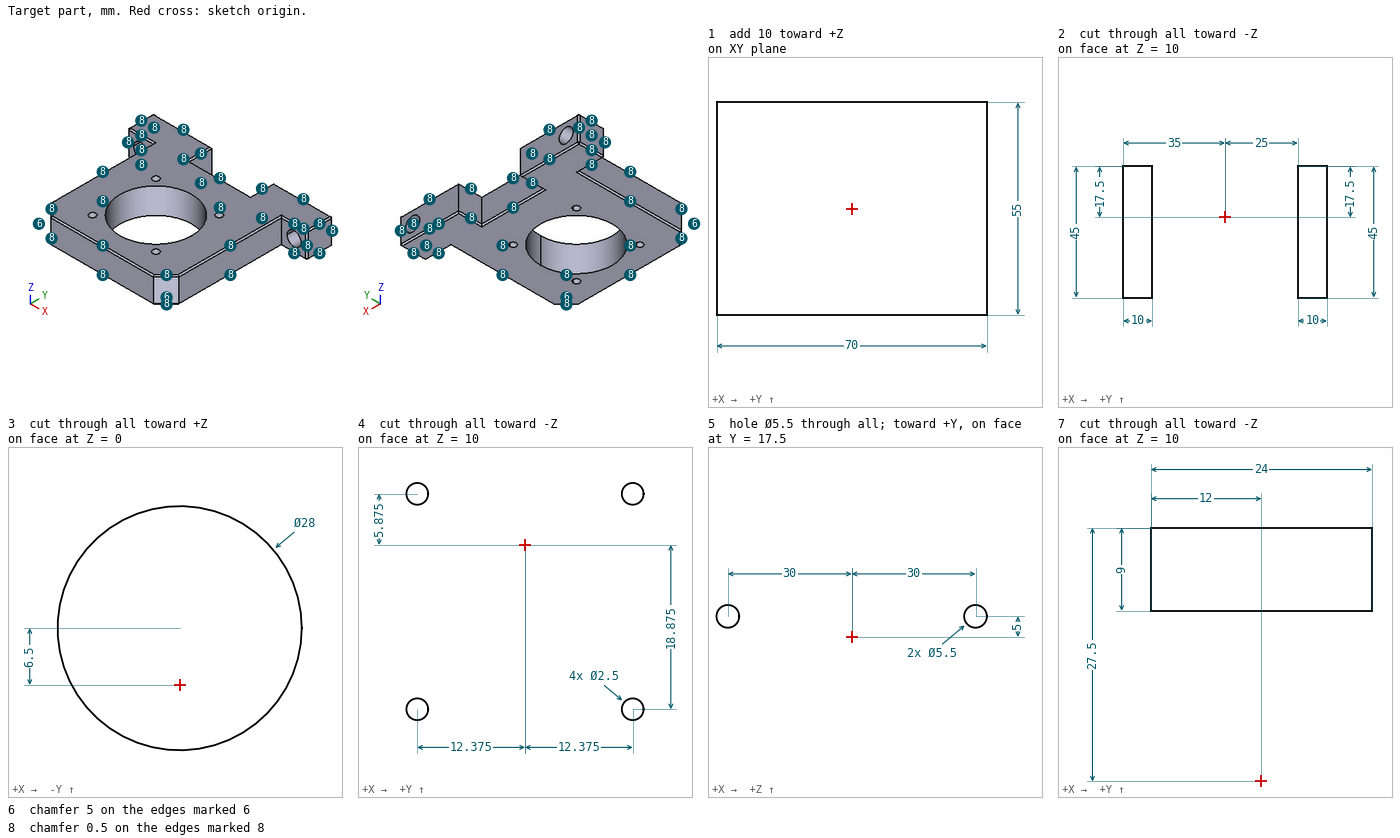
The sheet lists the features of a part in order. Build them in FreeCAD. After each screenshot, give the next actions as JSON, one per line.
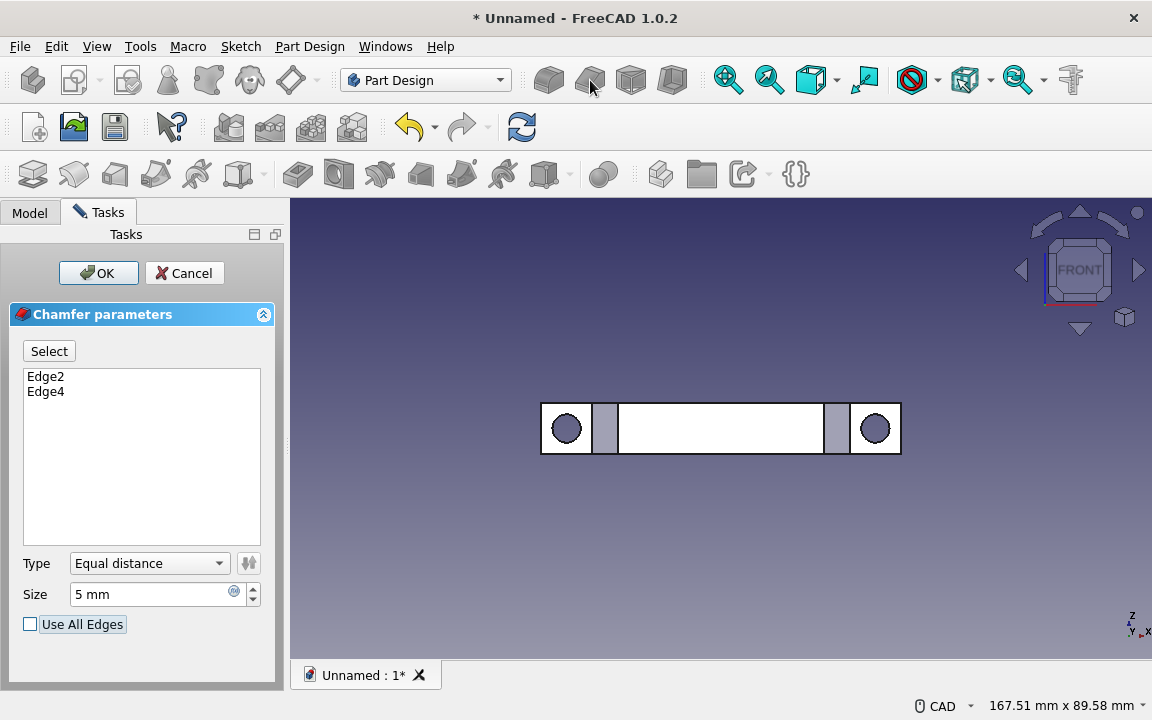
{"action": "left_click", "coordinate": [99, 273]}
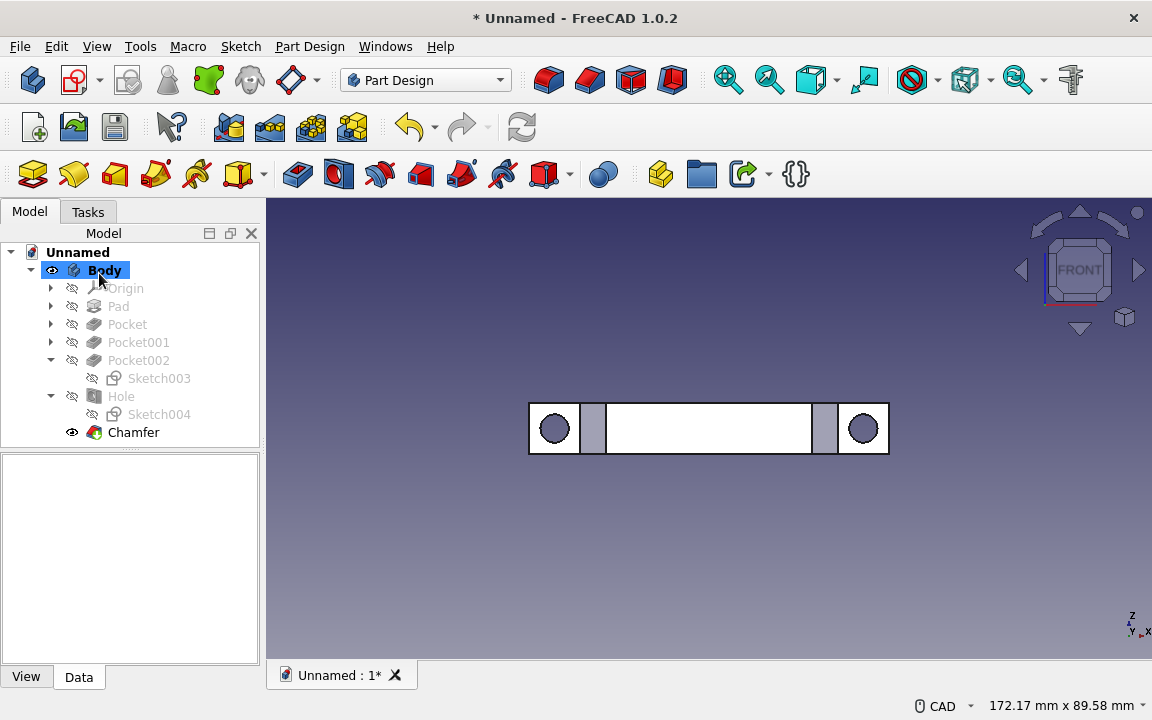
{"action": "key", "text": "v f"}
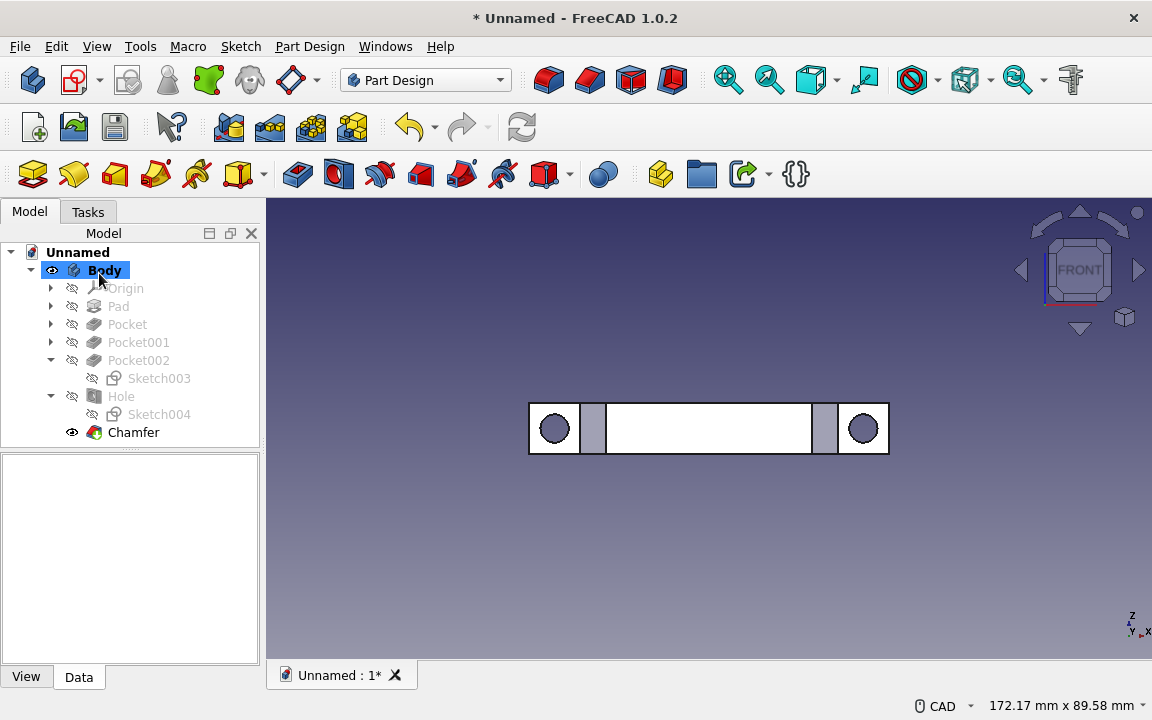
{"action": "key", "text": "0"}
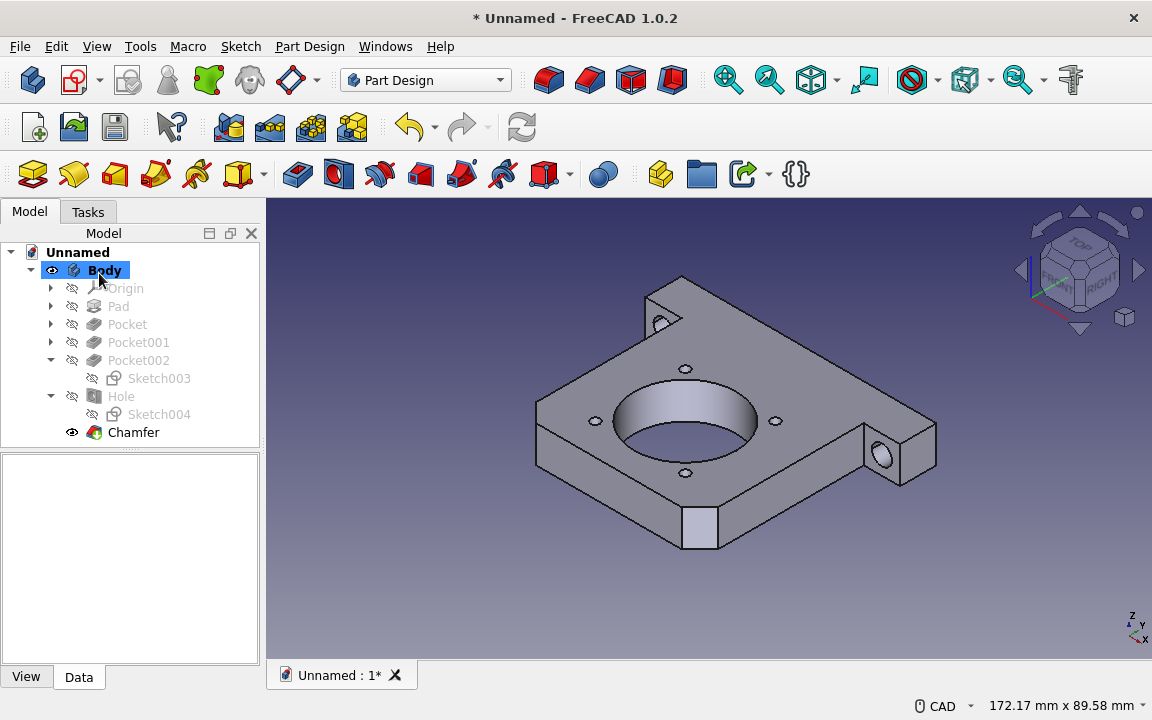
{"action": "left_click", "coordinate": [803, 394]}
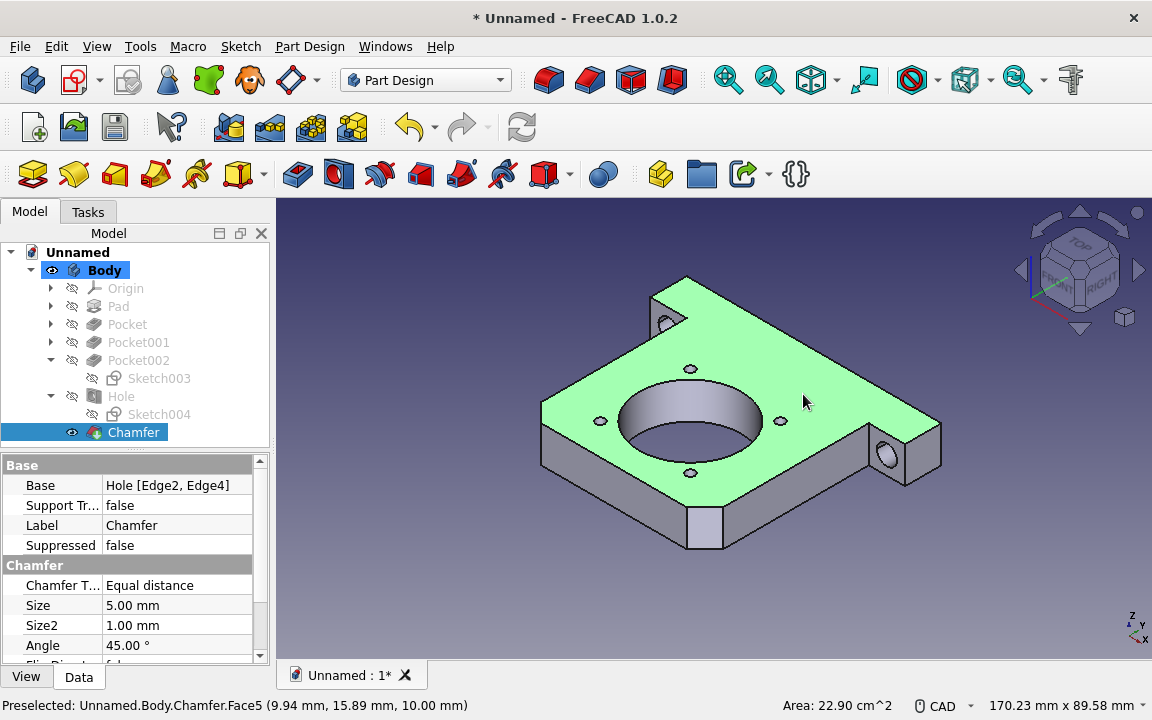
{"action": "left_click", "coordinate": [74, 80]}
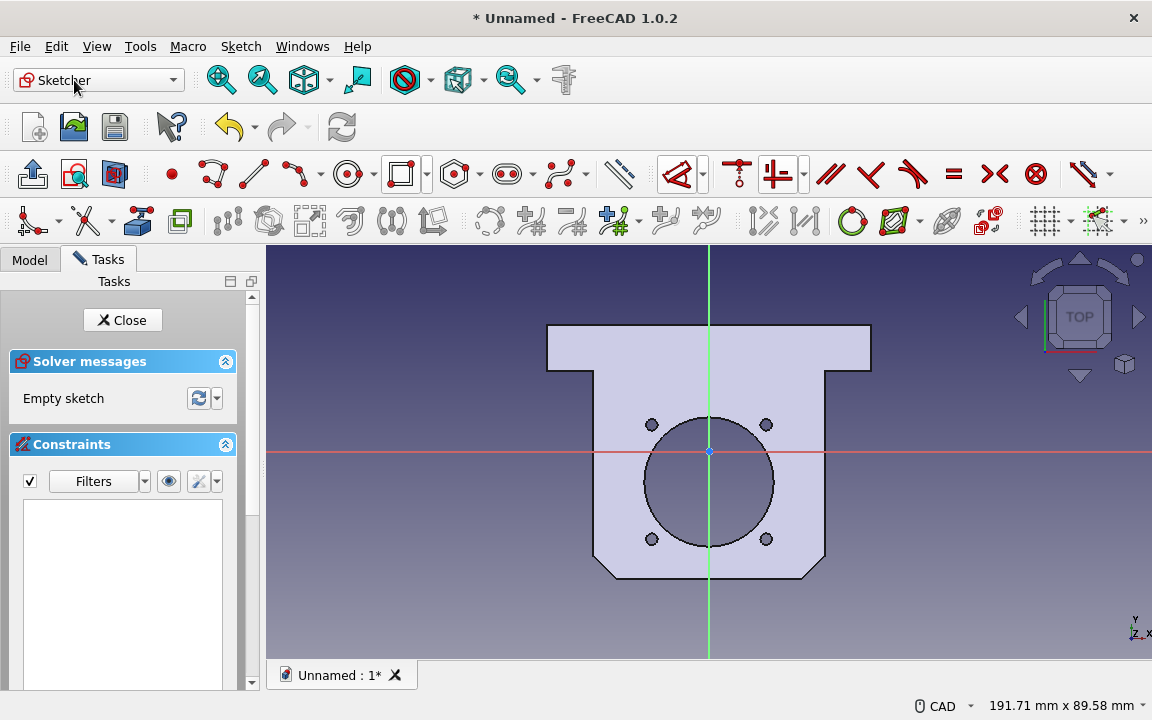
{"action": "scroll", "coordinate": [792, 311], "scroll_direction": "up", "scroll_amount": 3}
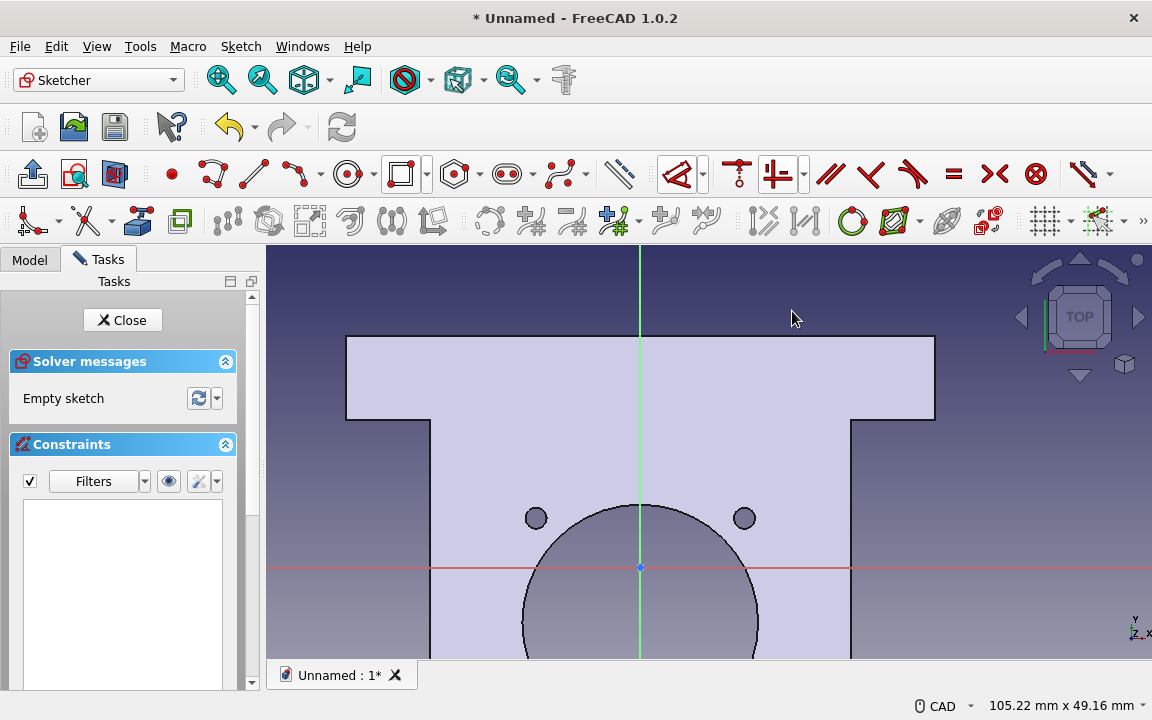
{"action": "left_click", "coordinate": [400, 174]}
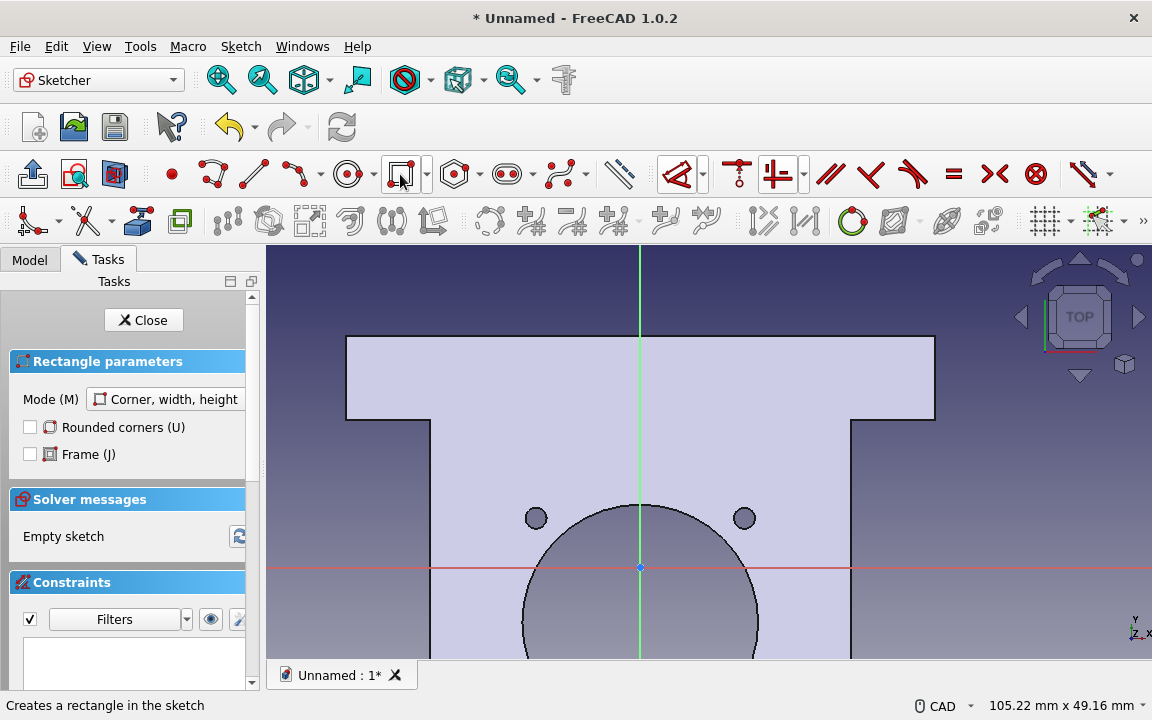
{"action": "left_click", "coordinate": [539, 336]}
{"action": "left_click", "coordinate": [741, 412]}
{"action": "key", "text": "Escape"}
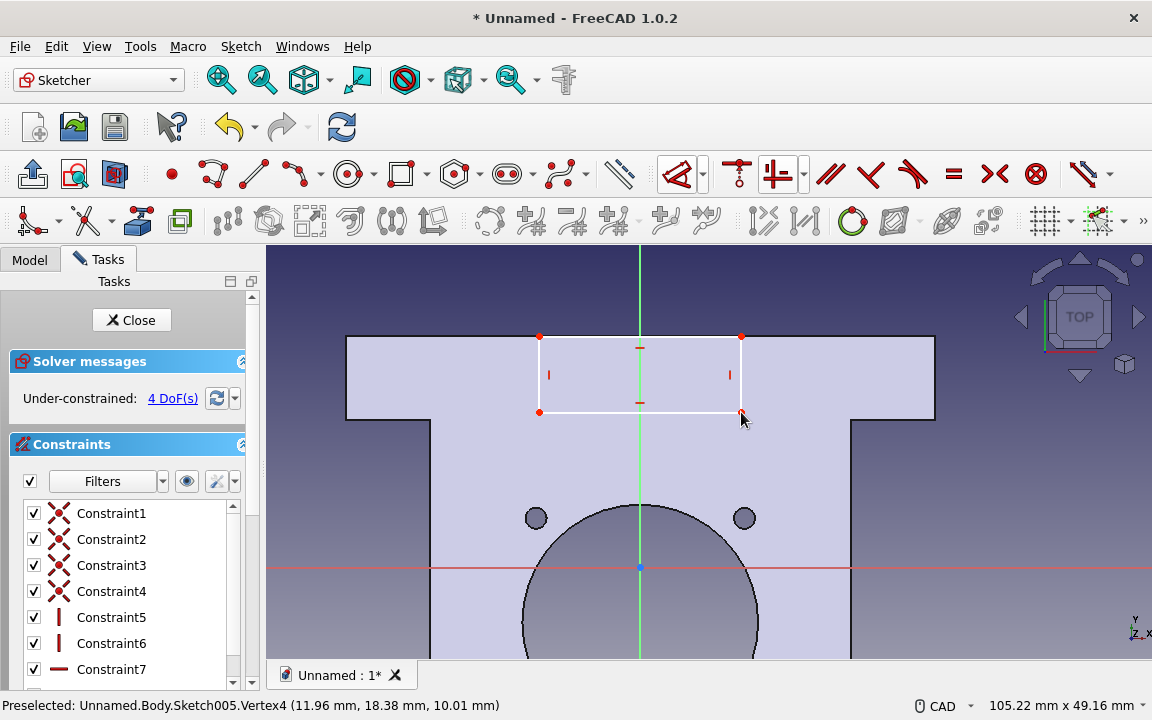
{"action": "left_click", "coordinate": [539, 360]}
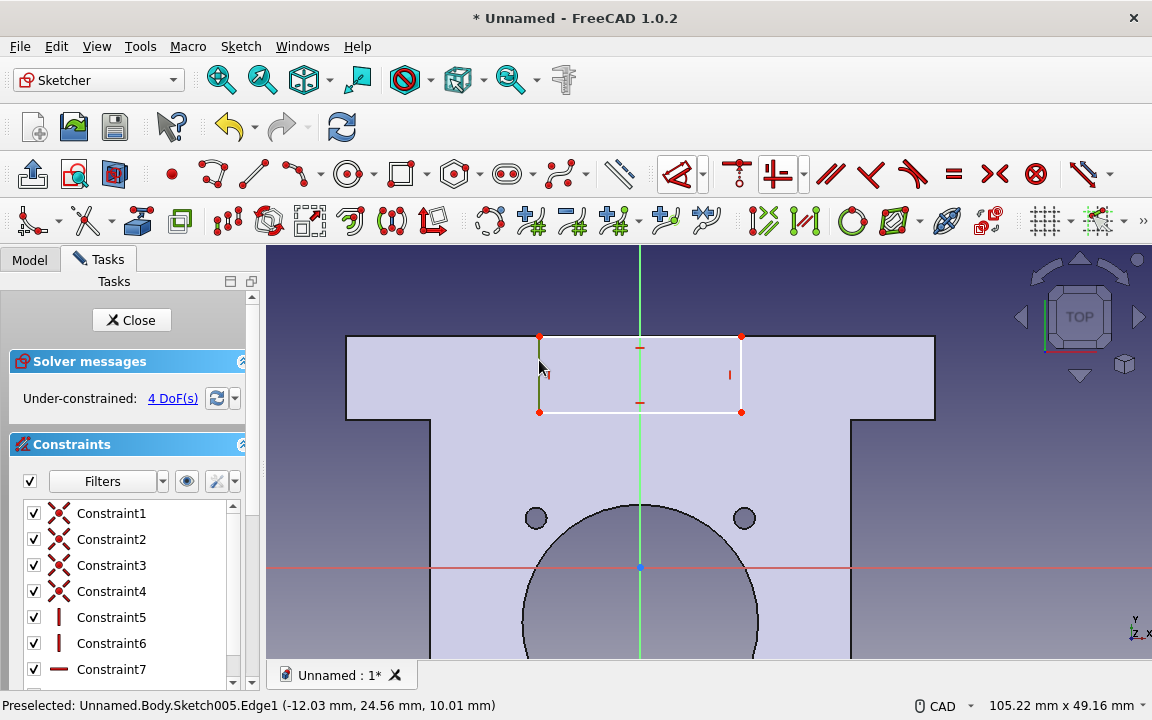
{"action": "key", "text": "i"}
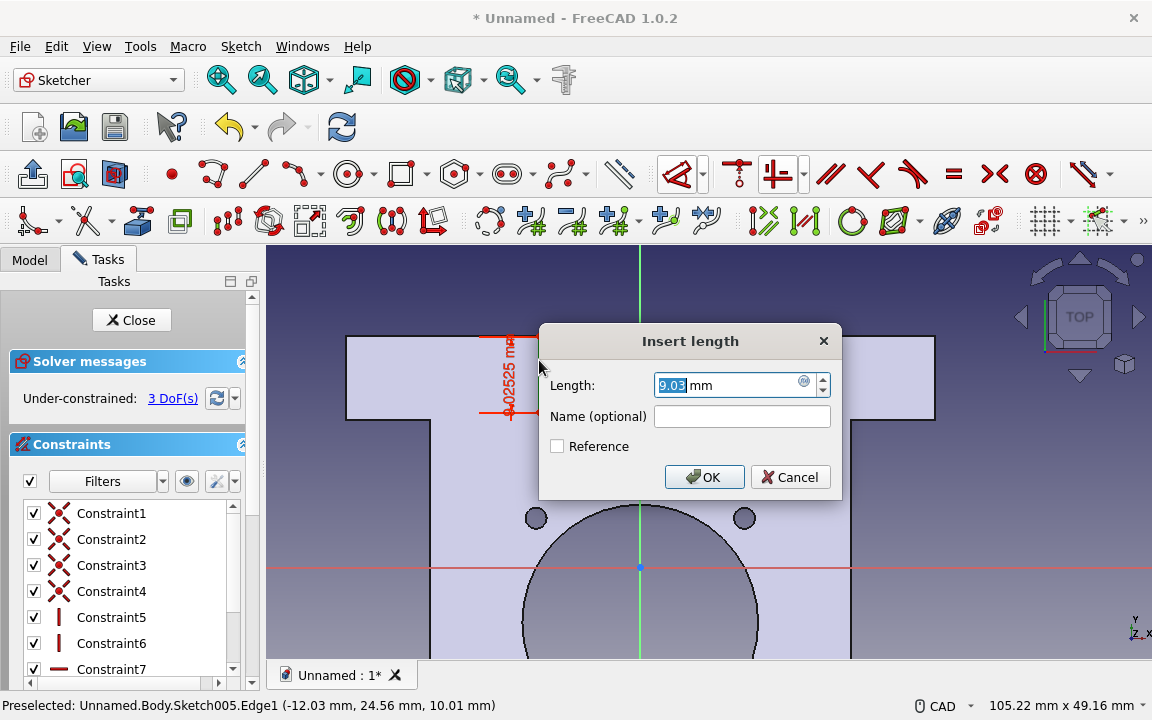
{"action": "type", "text": "9"}
{"action": "key", "text": "Return"}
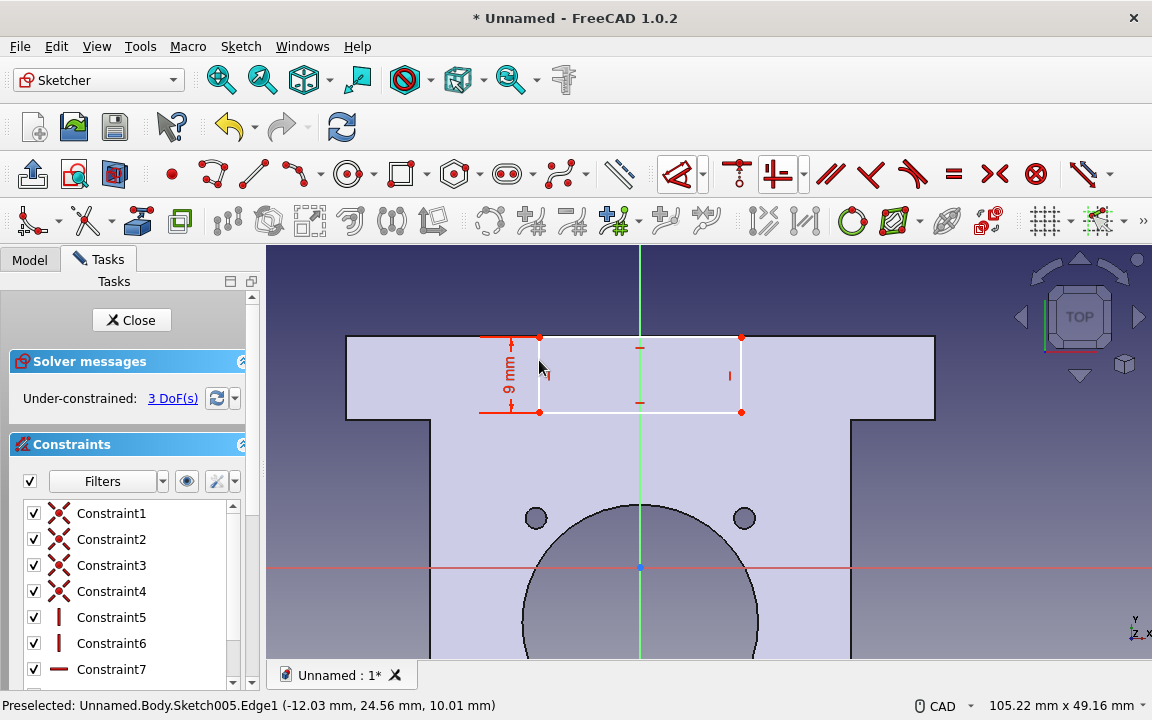
{"action": "left_click", "coordinate": [600, 413]}